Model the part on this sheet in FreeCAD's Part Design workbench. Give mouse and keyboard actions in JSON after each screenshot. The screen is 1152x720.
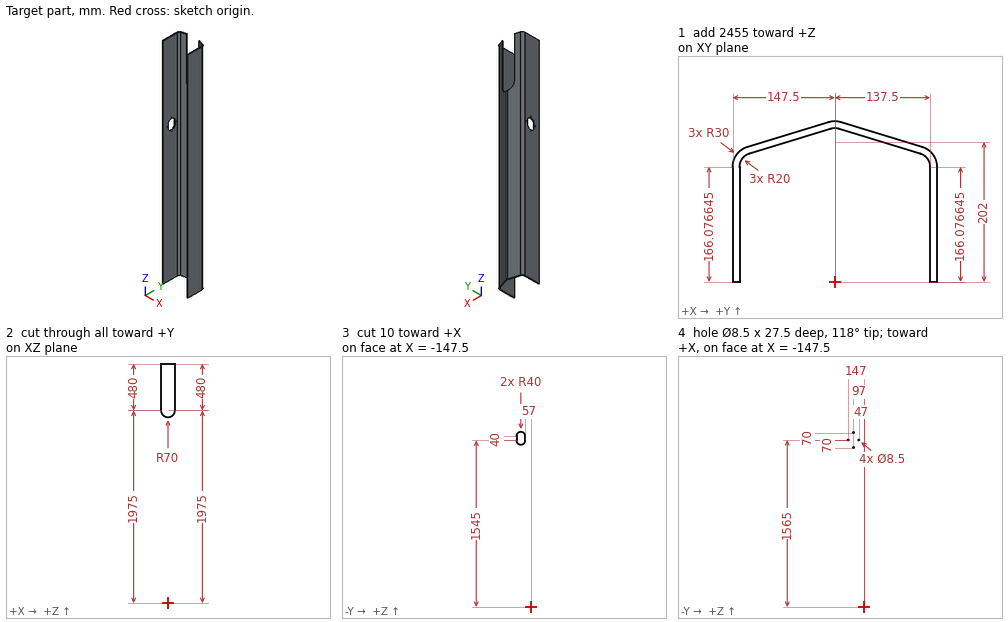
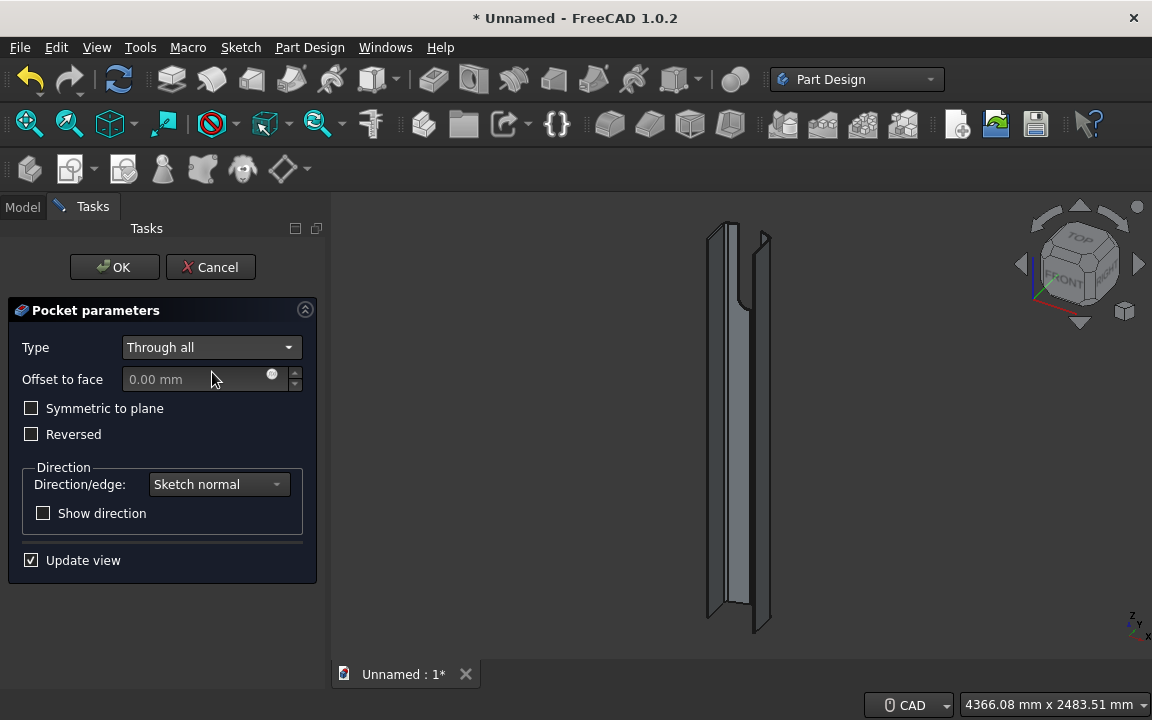
{"action": "left_click", "coordinate": [115, 267]}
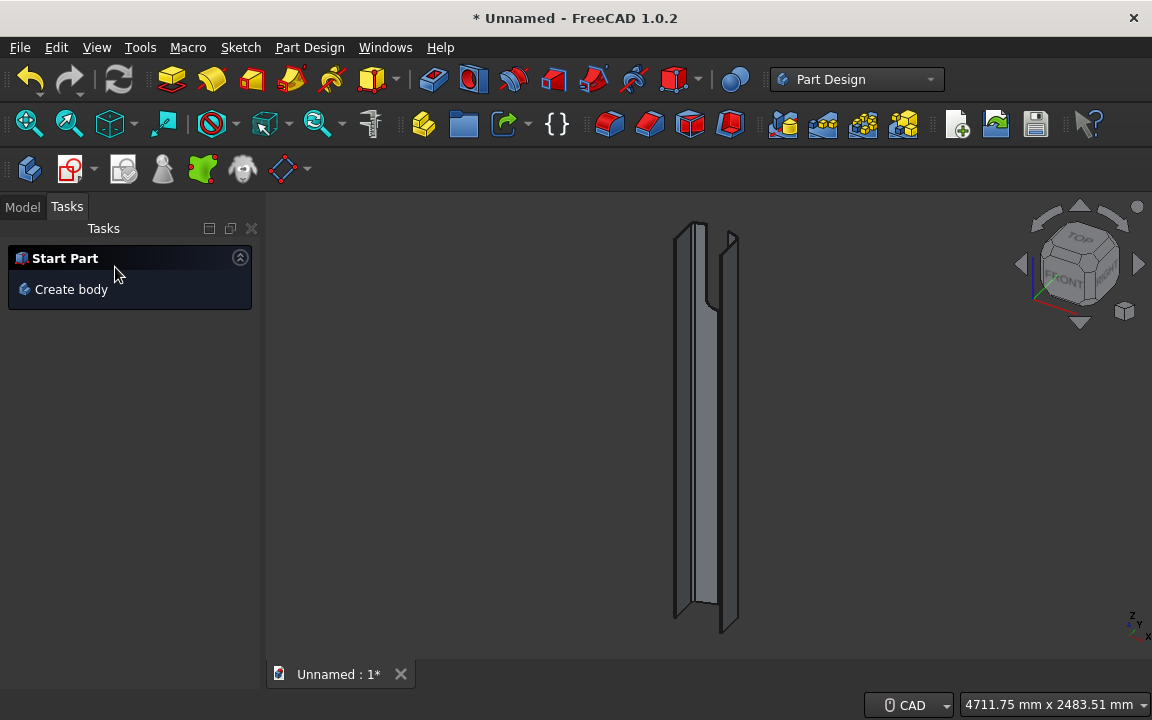
{"action": "key", "text": "6"}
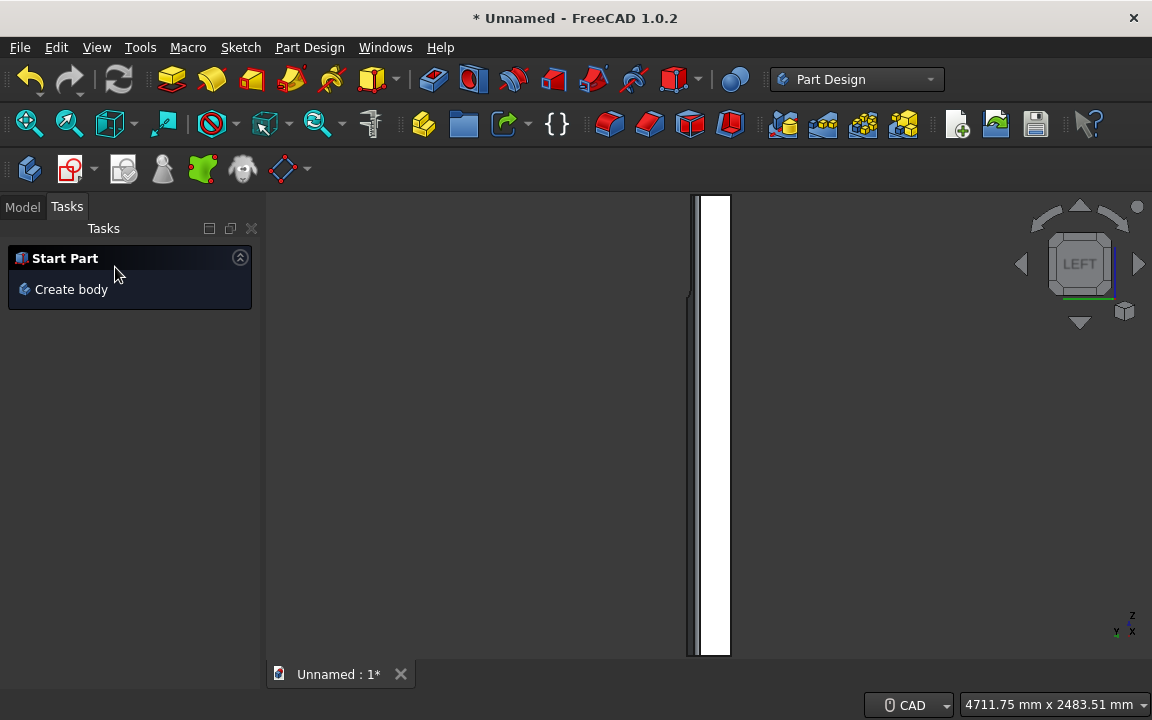
{"action": "left_click", "coordinate": [715, 227]}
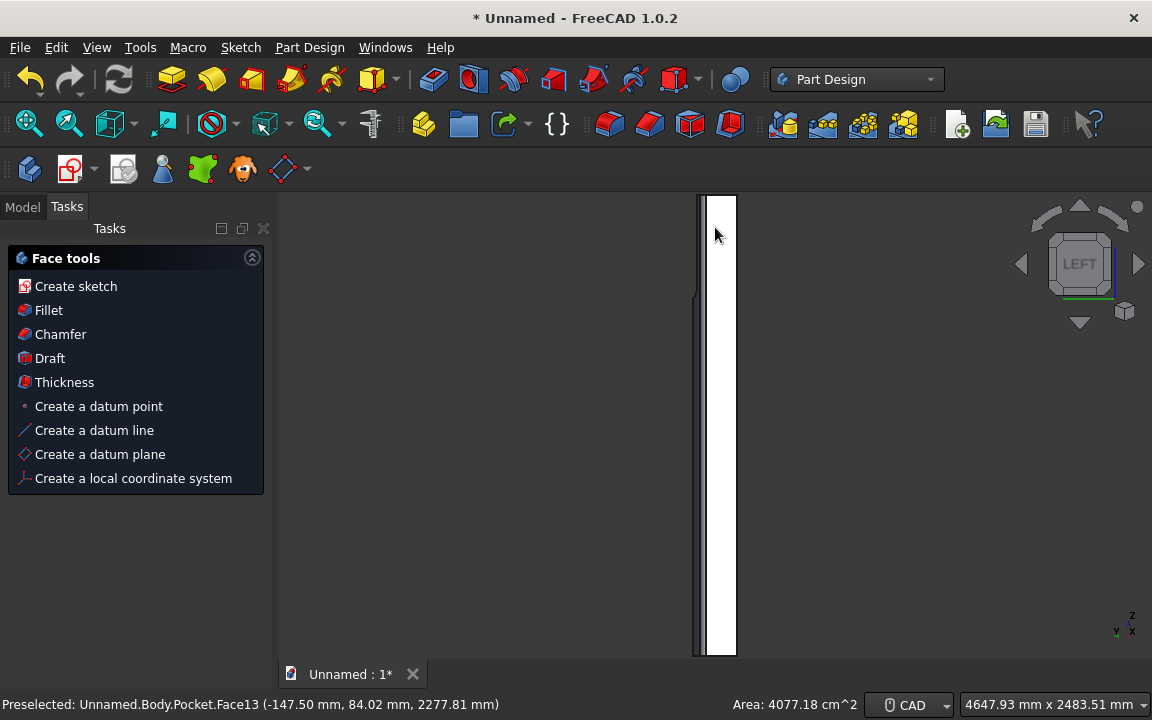
{"action": "left_click", "coordinate": [70, 170]}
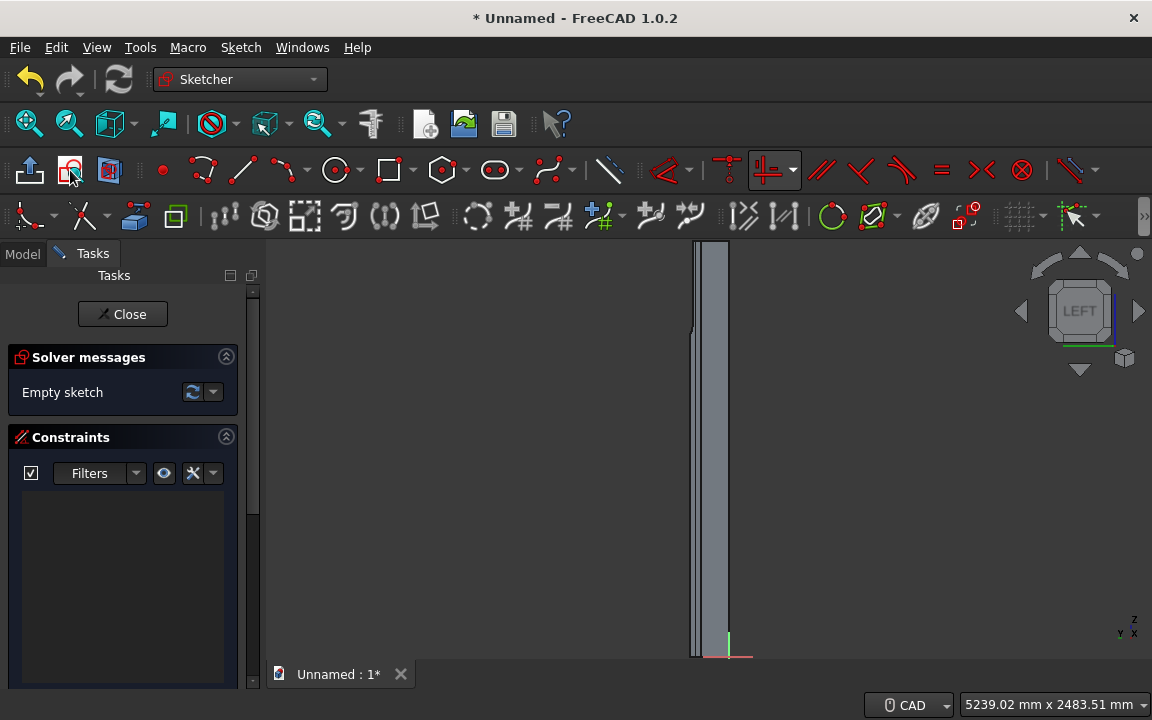
{"action": "scroll", "coordinate": [718, 387], "scroll_direction": "up", "scroll_amount": 13}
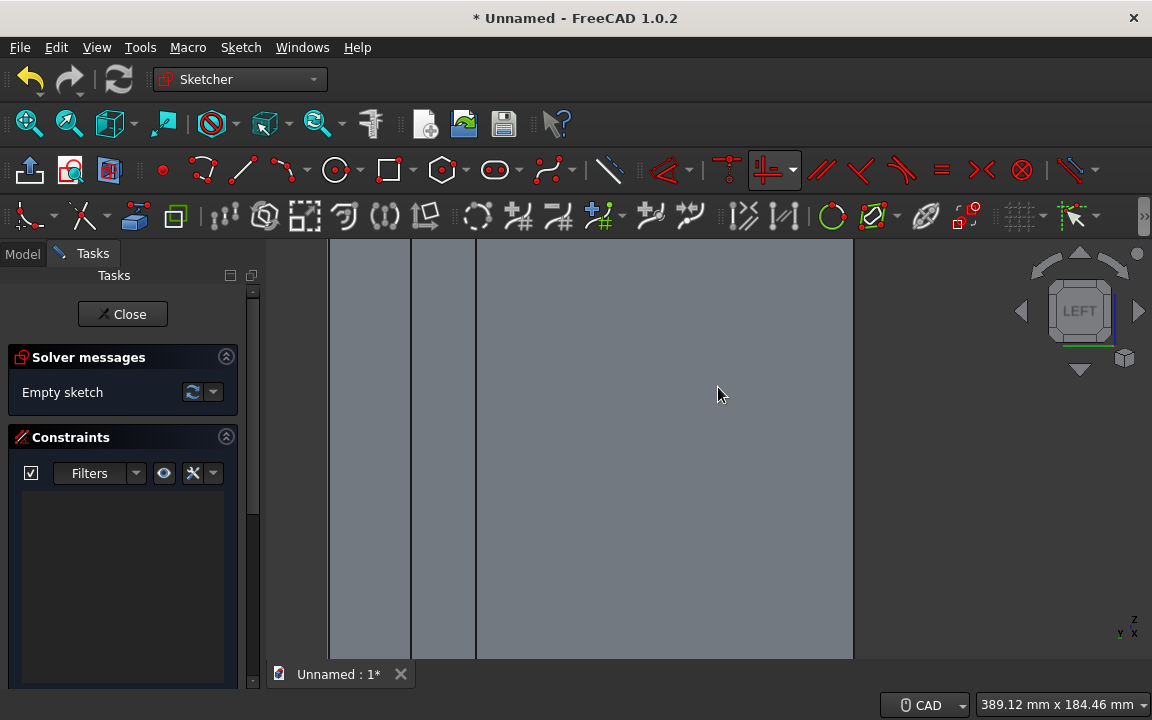
{"action": "left_click", "coordinate": [496, 170]}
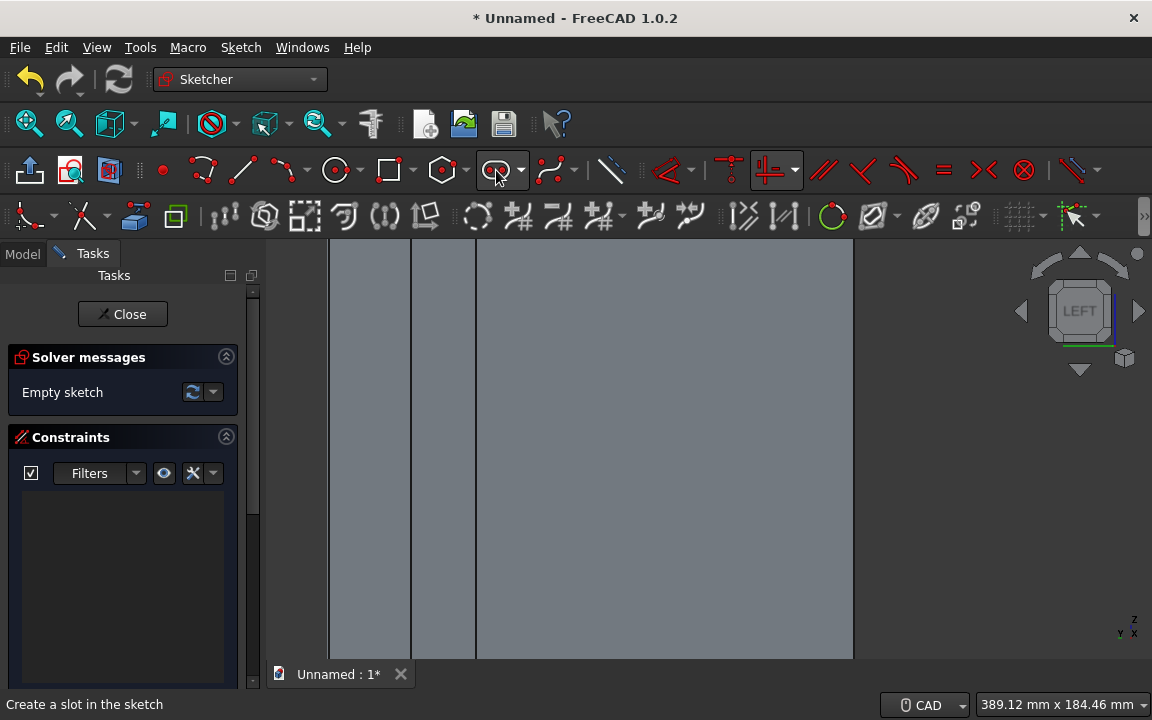
{"action": "left_click", "coordinate": [634, 494]}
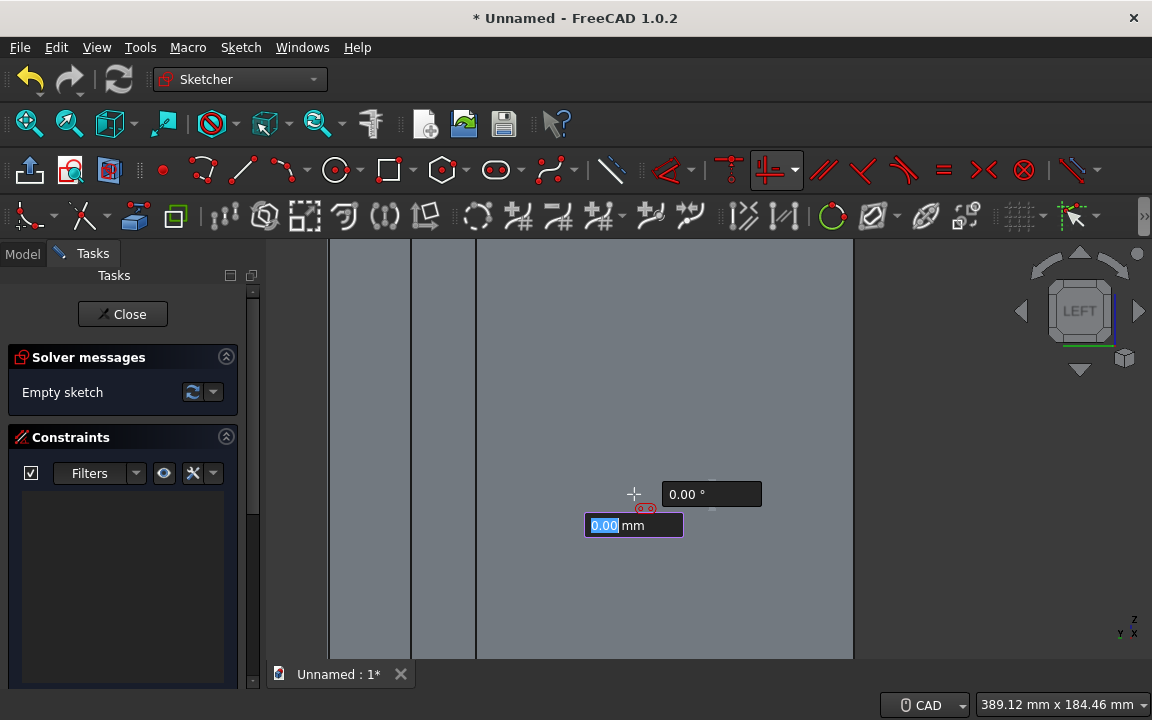
{"action": "left_click", "coordinate": [634, 403]}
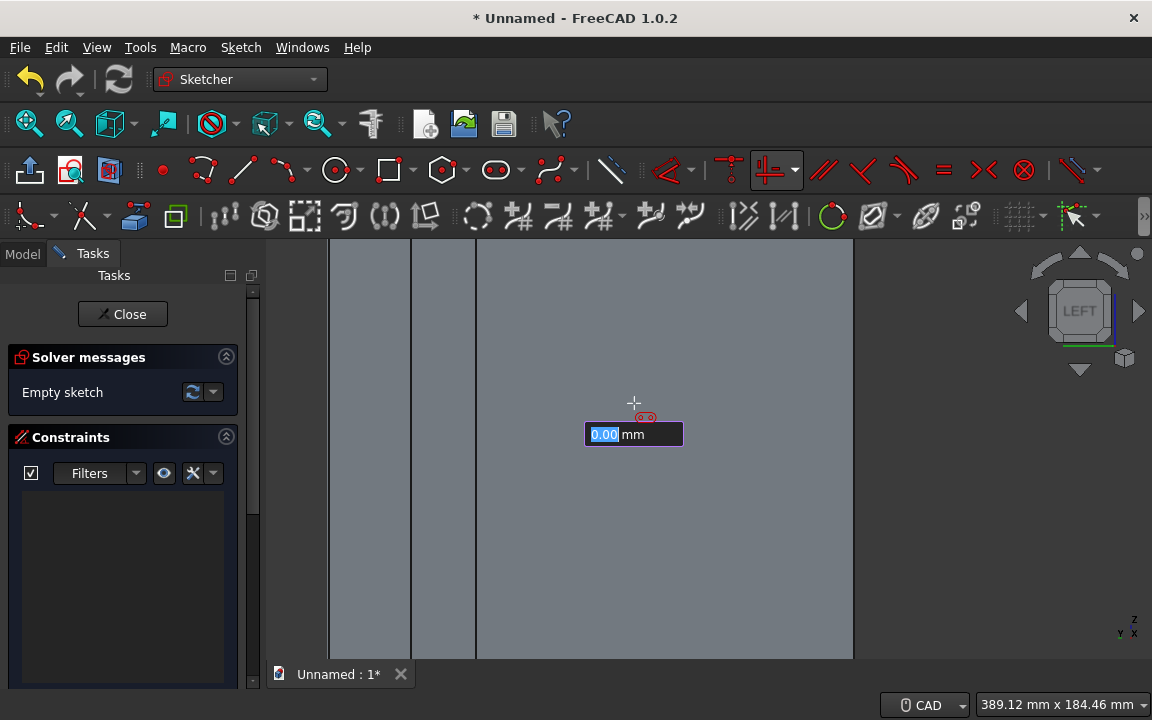
{"action": "left_click", "coordinate": [542, 449]}
{"action": "key", "text": "Escape"}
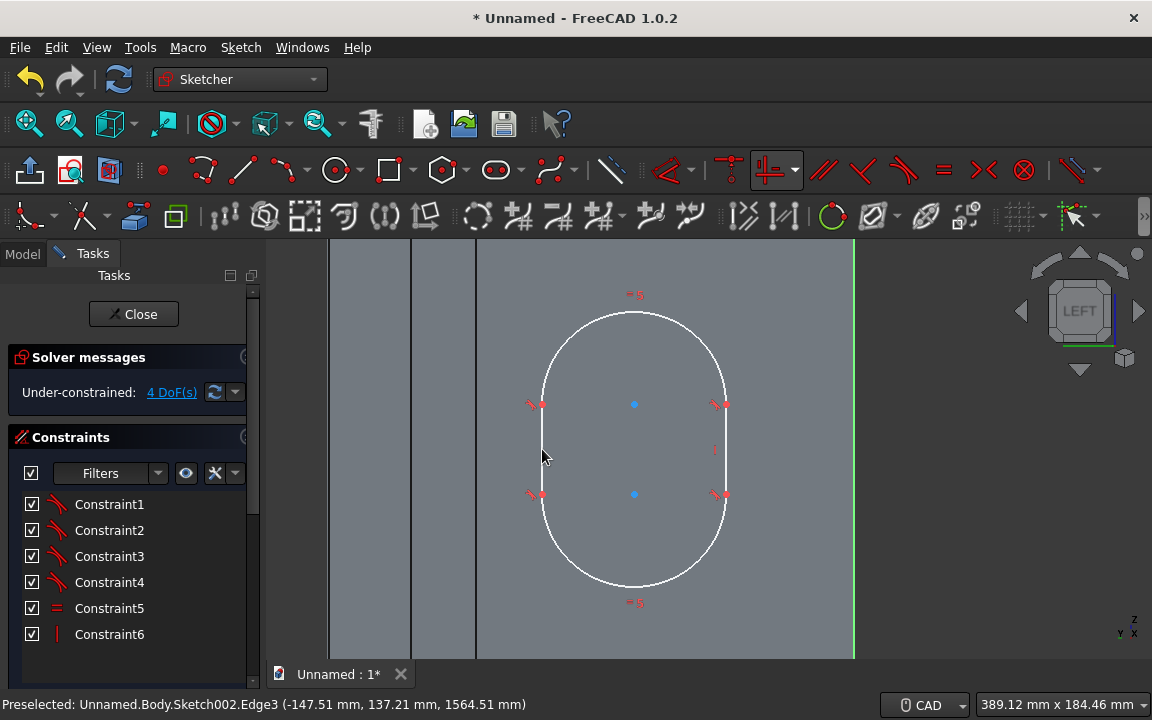
{"action": "left_click", "coordinate": [666, 170]}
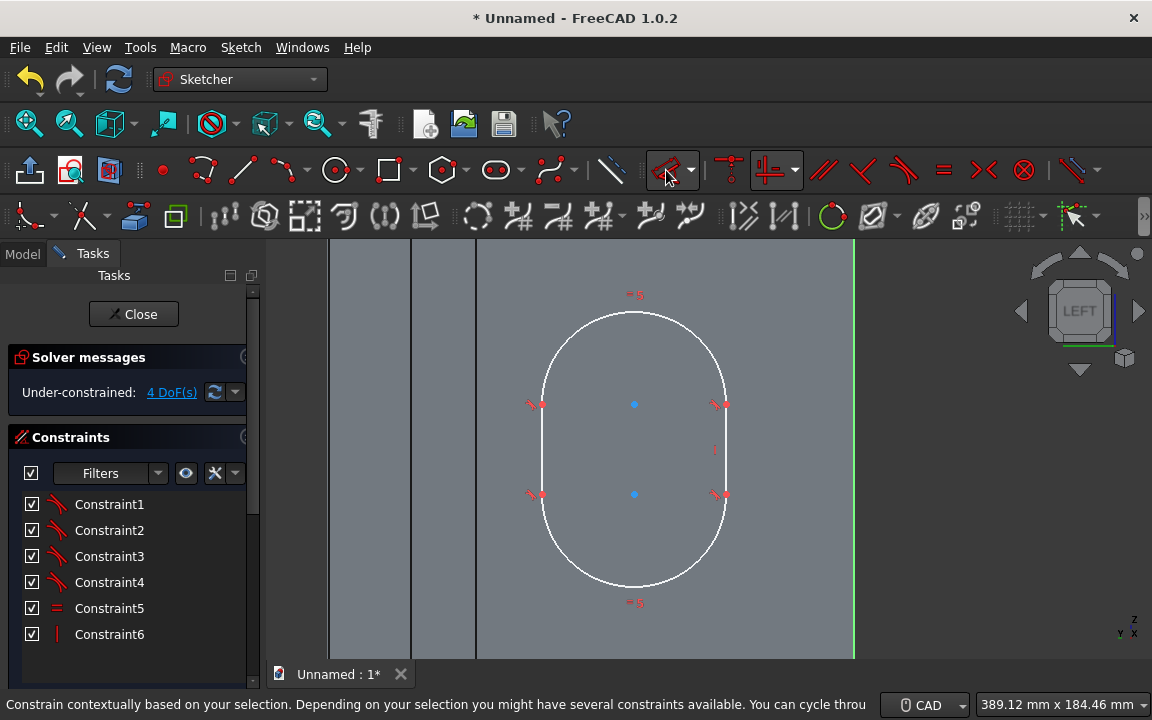
{"action": "left_click", "coordinate": [580, 569]}
{"action": "left_click", "coordinate": [561, 595]}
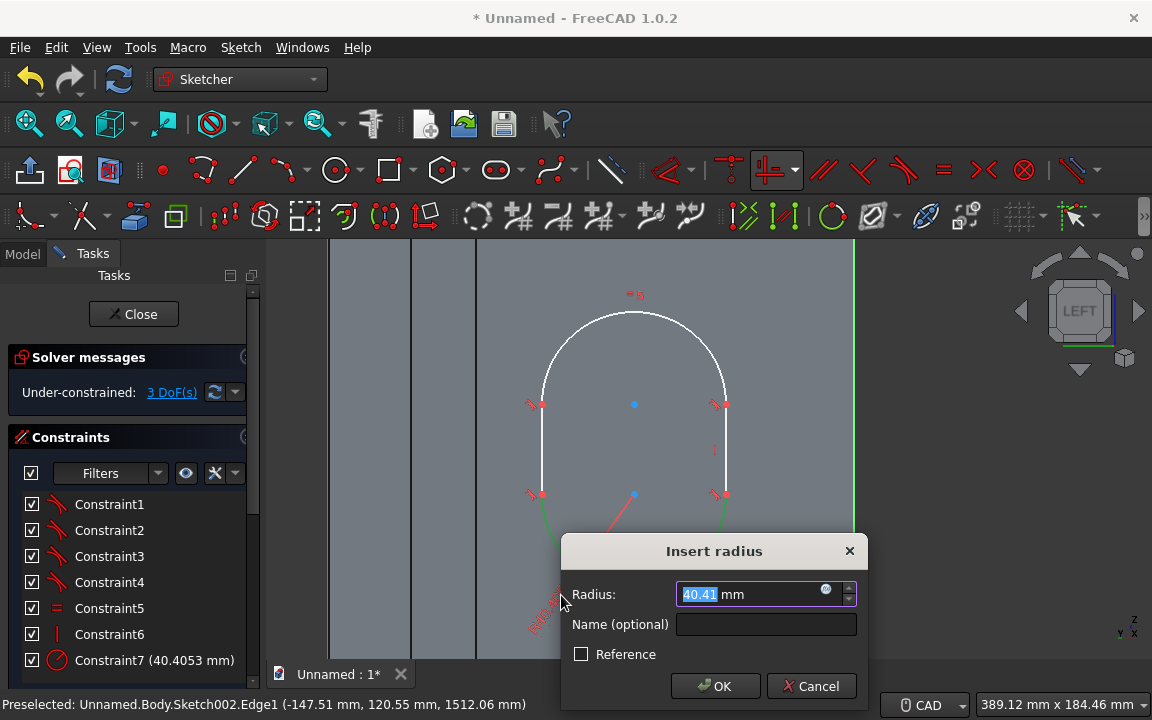
{"action": "type", "text": "40"}
{"action": "key", "text": "Return"}